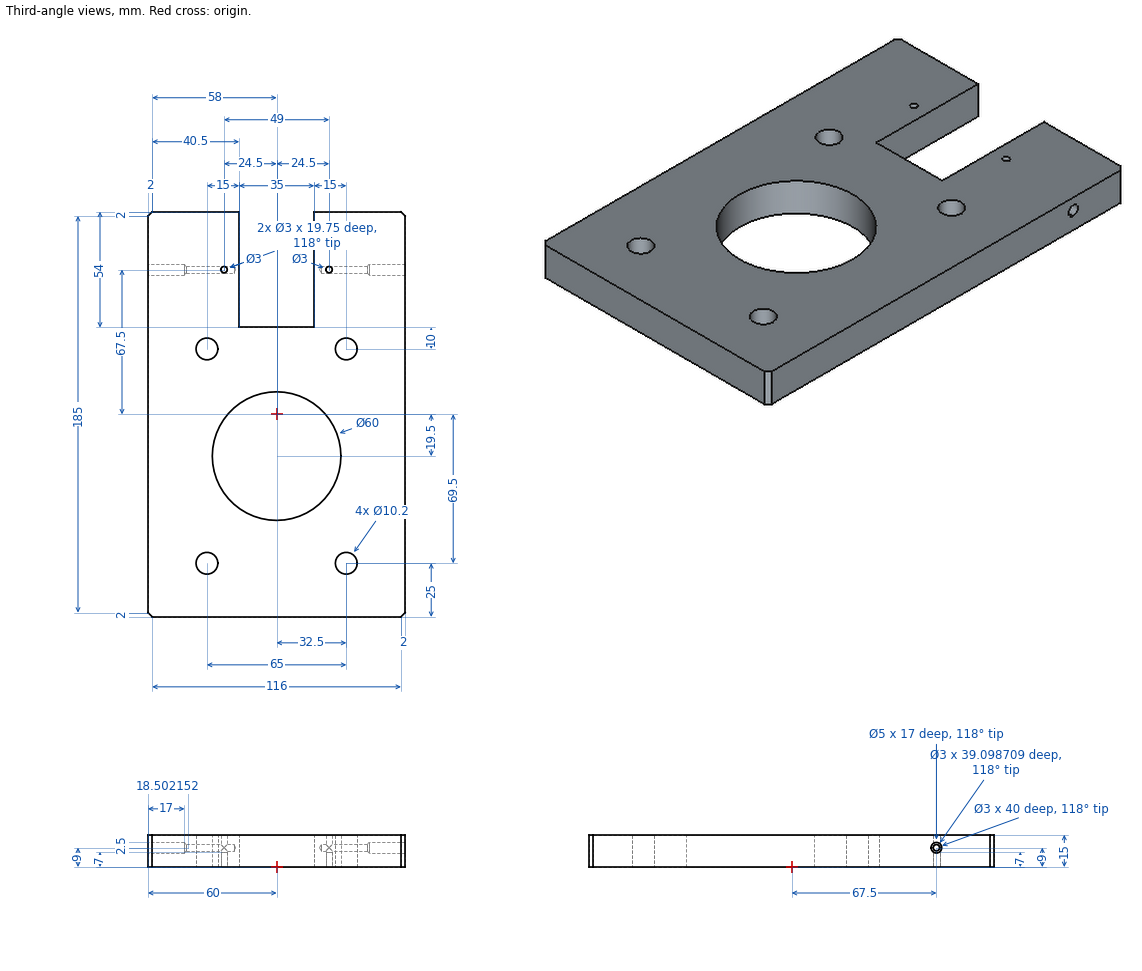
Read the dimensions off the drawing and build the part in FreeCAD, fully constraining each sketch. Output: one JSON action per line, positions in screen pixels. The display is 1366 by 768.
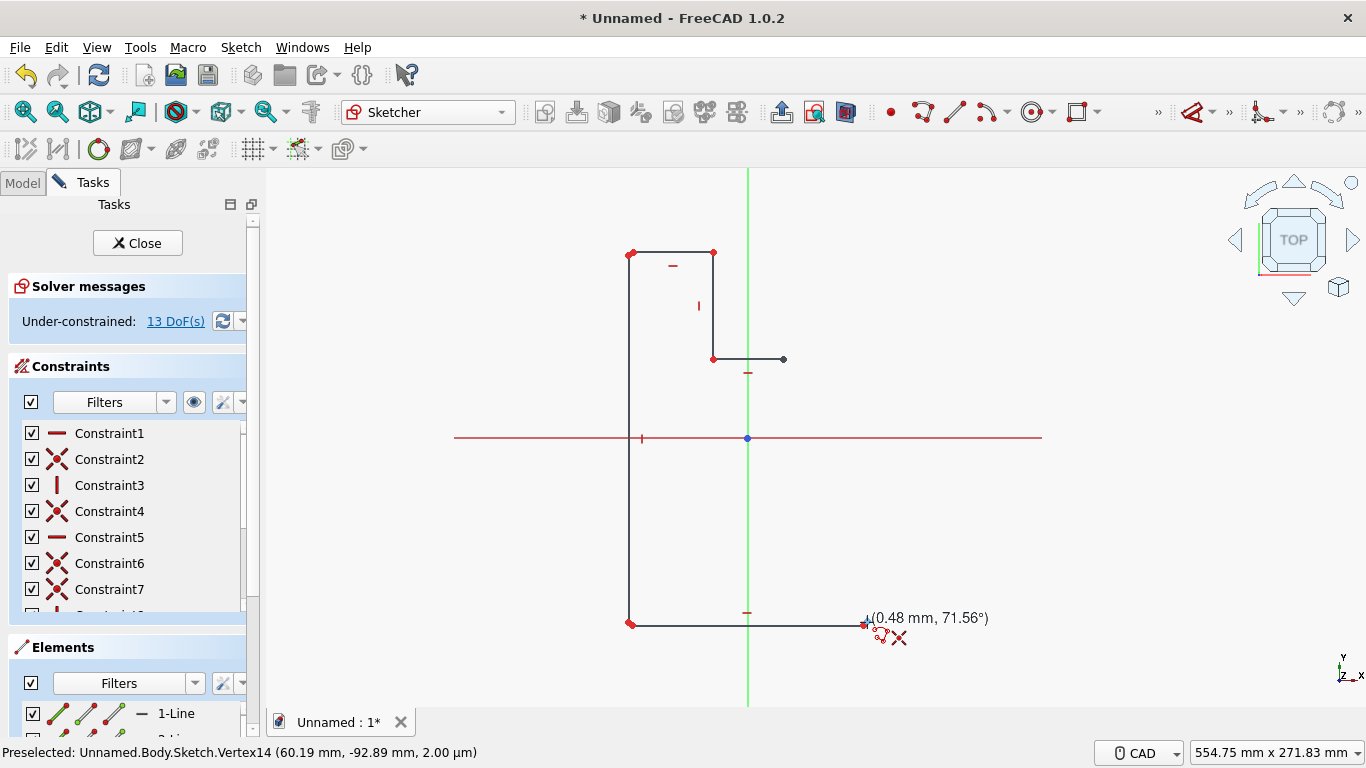
{"action": "left_click", "coordinate": [867, 255]}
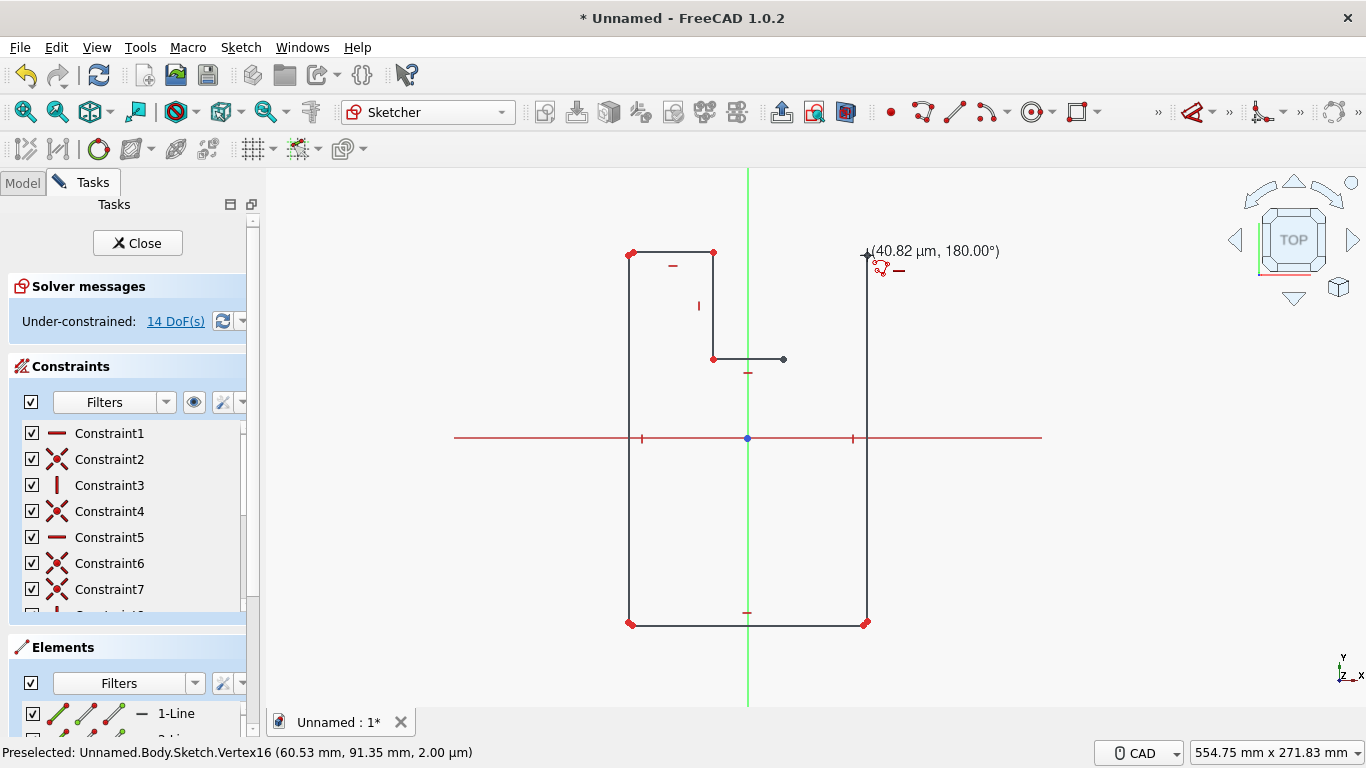
{"action": "scroll", "coordinate": [863, 251], "scroll_direction": "up", "scroll_amount": 6}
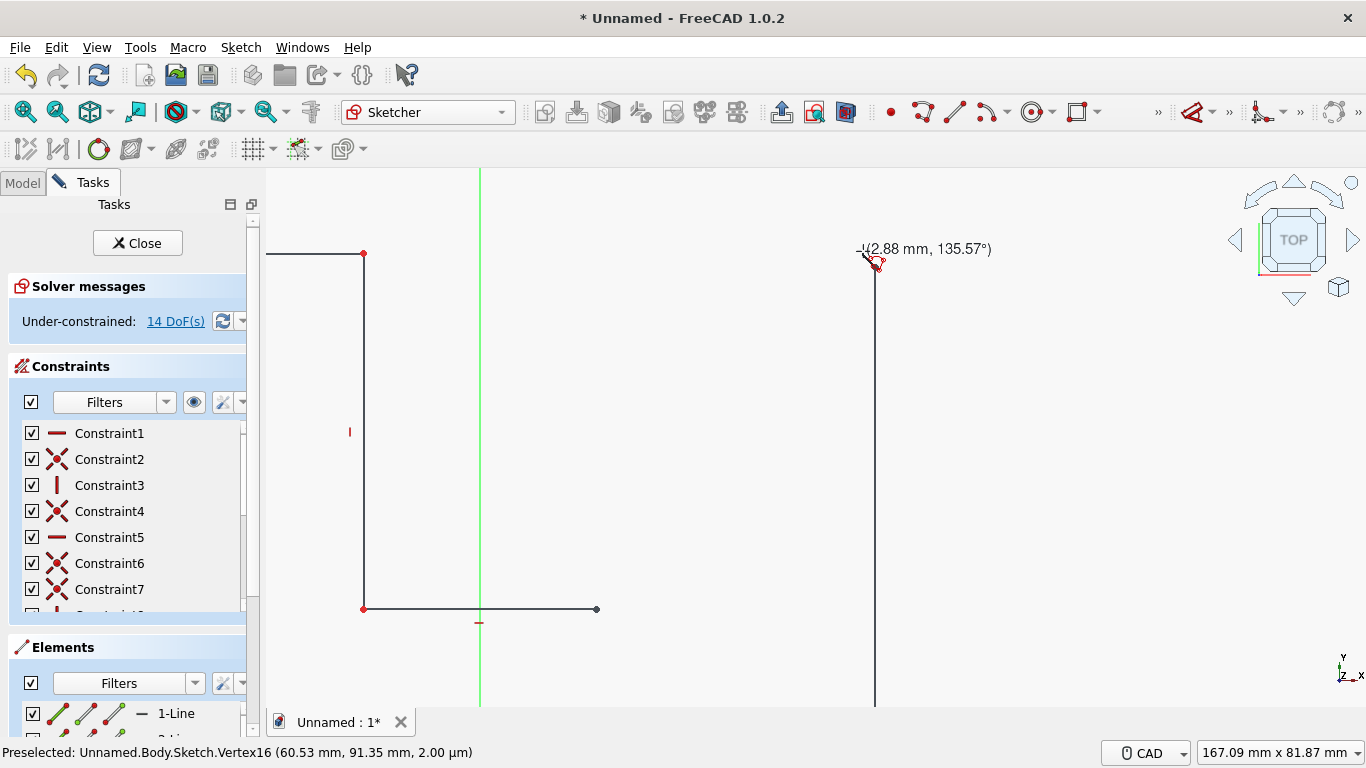
{"action": "left_click", "coordinate": [862, 250]}
{"action": "left_click", "coordinate": [595, 250]}
{"action": "left_click", "coordinate": [596, 609]}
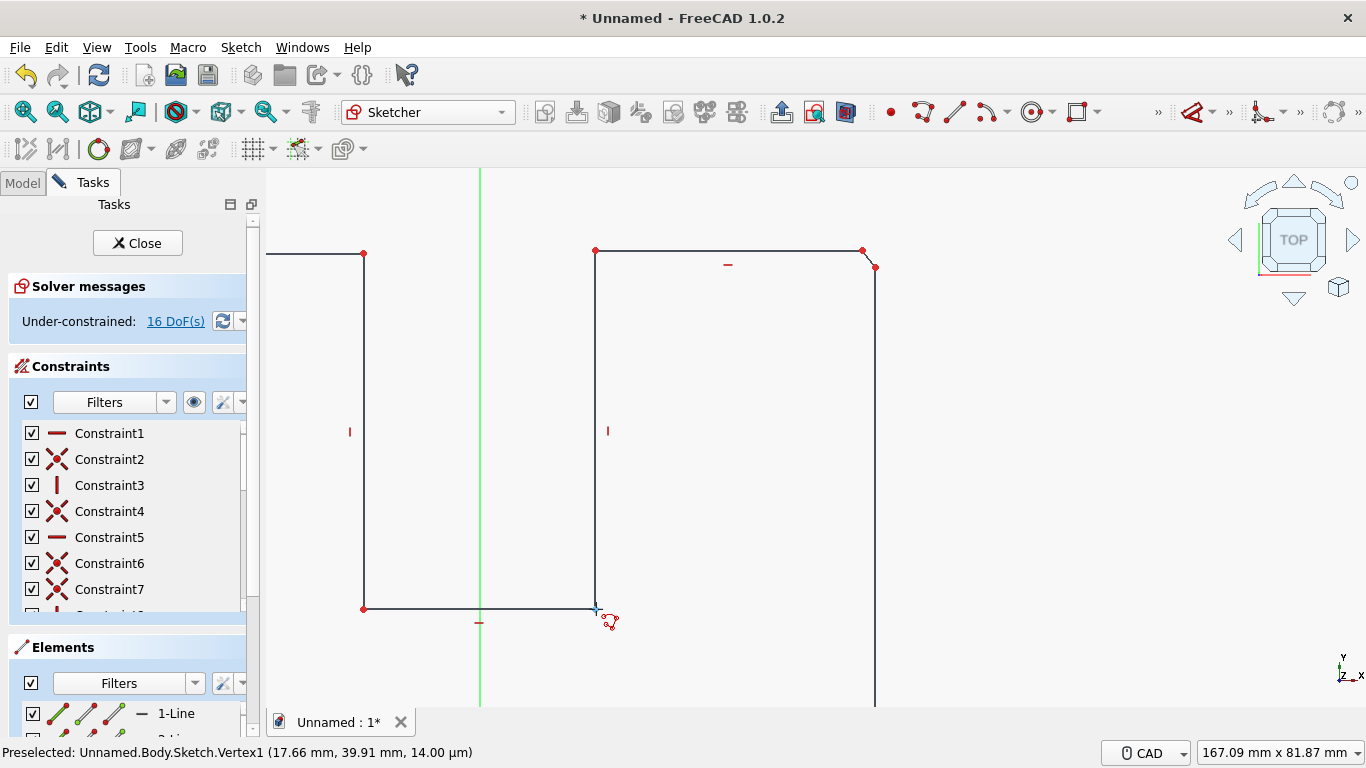
{"action": "left_click", "coordinate": [1032, 112]}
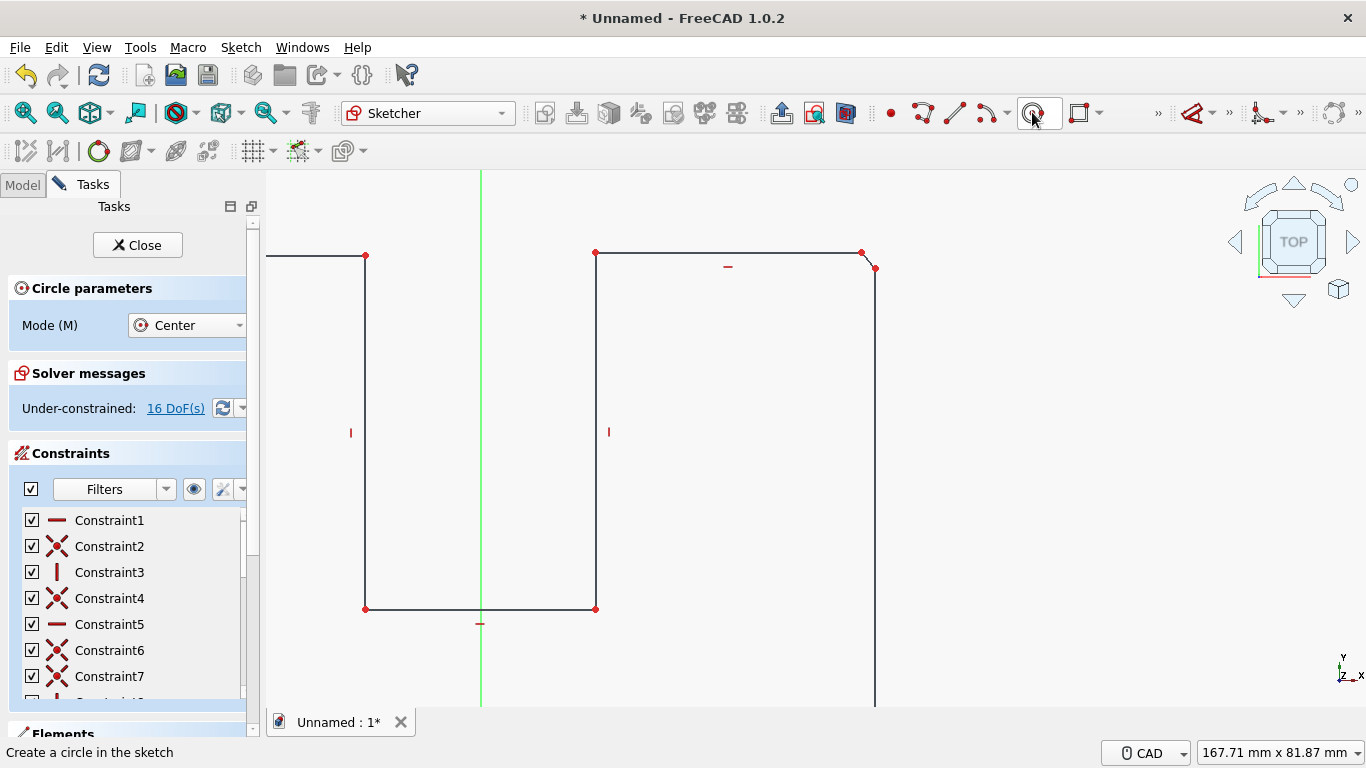
{"action": "scroll", "coordinate": [862, 252], "scroll_direction": "down", "scroll_amount": 6}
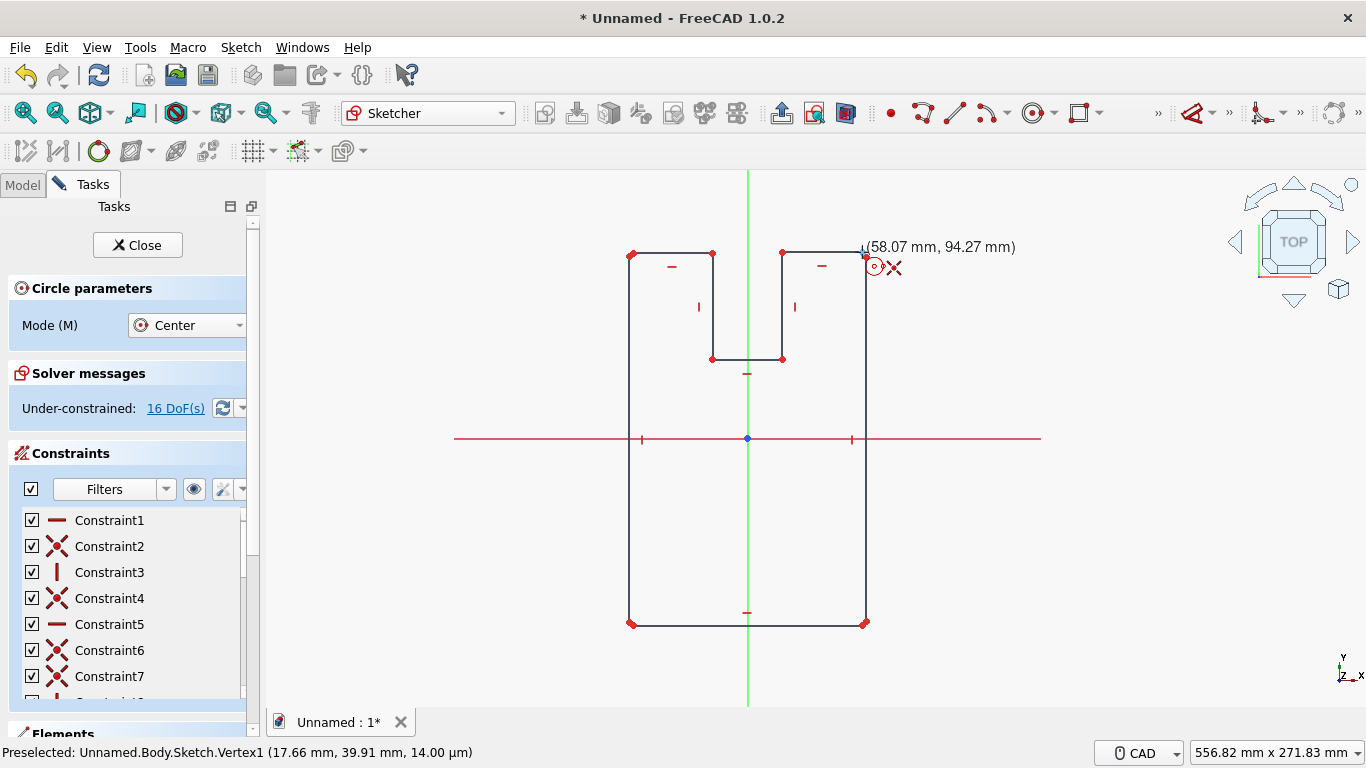
{"action": "scroll", "coordinate": [812, 576], "scroll_direction": "up", "scroll_amount": 5}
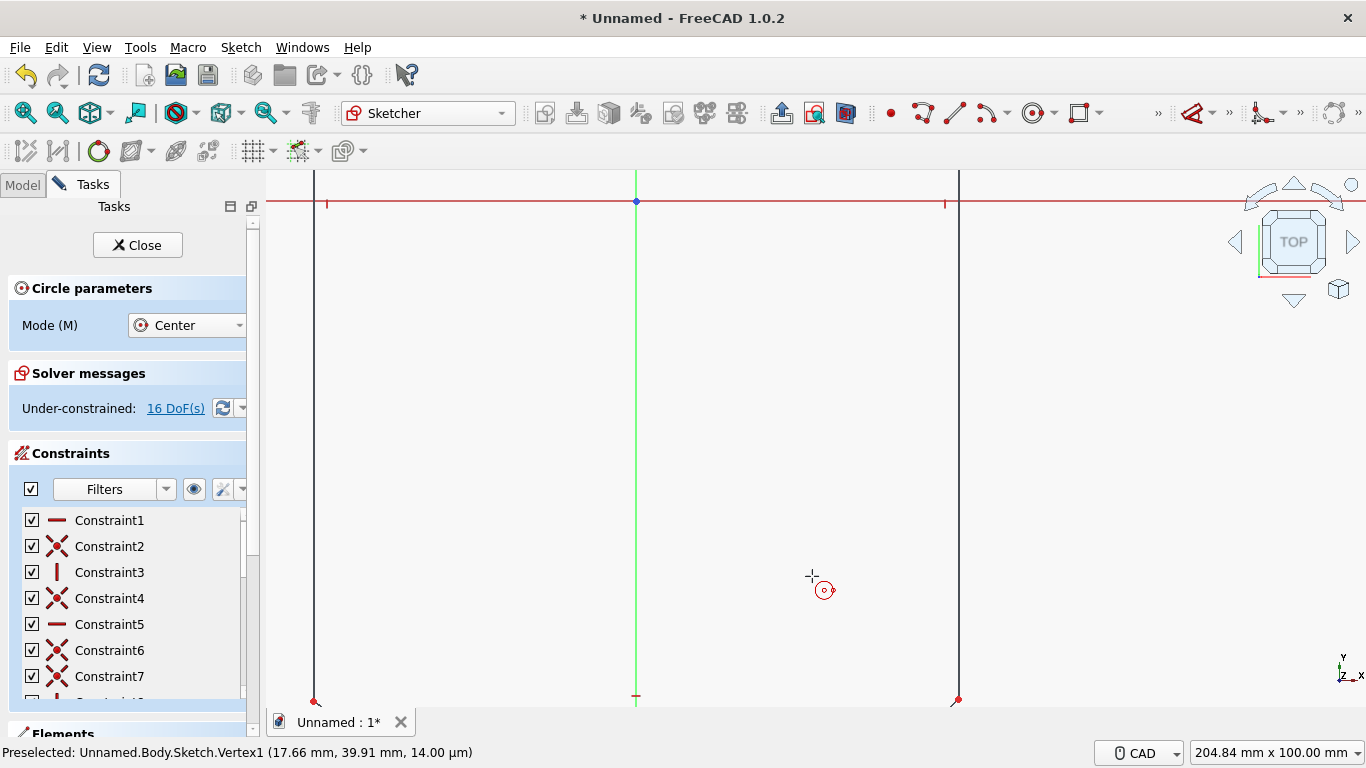
{"action": "left_click", "coordinate": [811, 575]}
{"action": "mouse_move", "coordinate": [830, 555]}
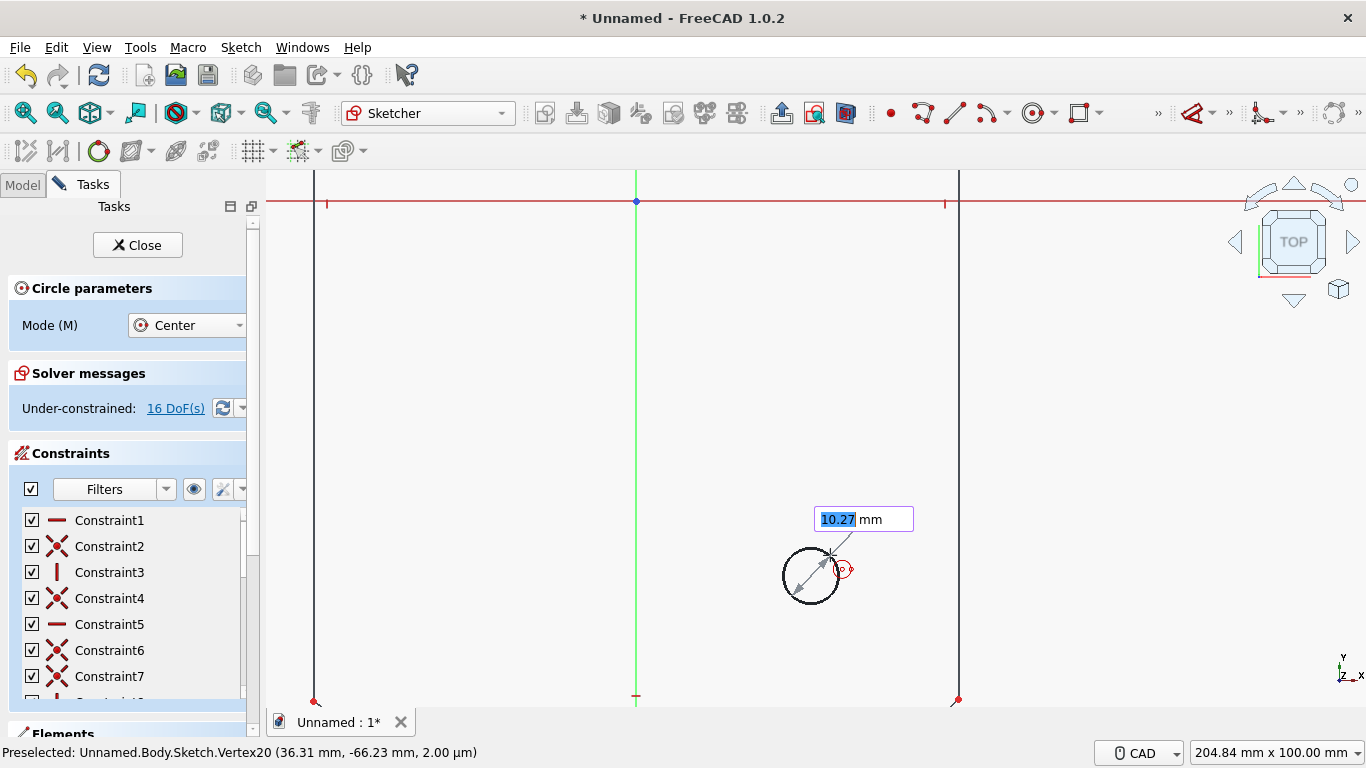
{"action": "type", "text": "10.2"}
{"action": "key", "text": "Return"}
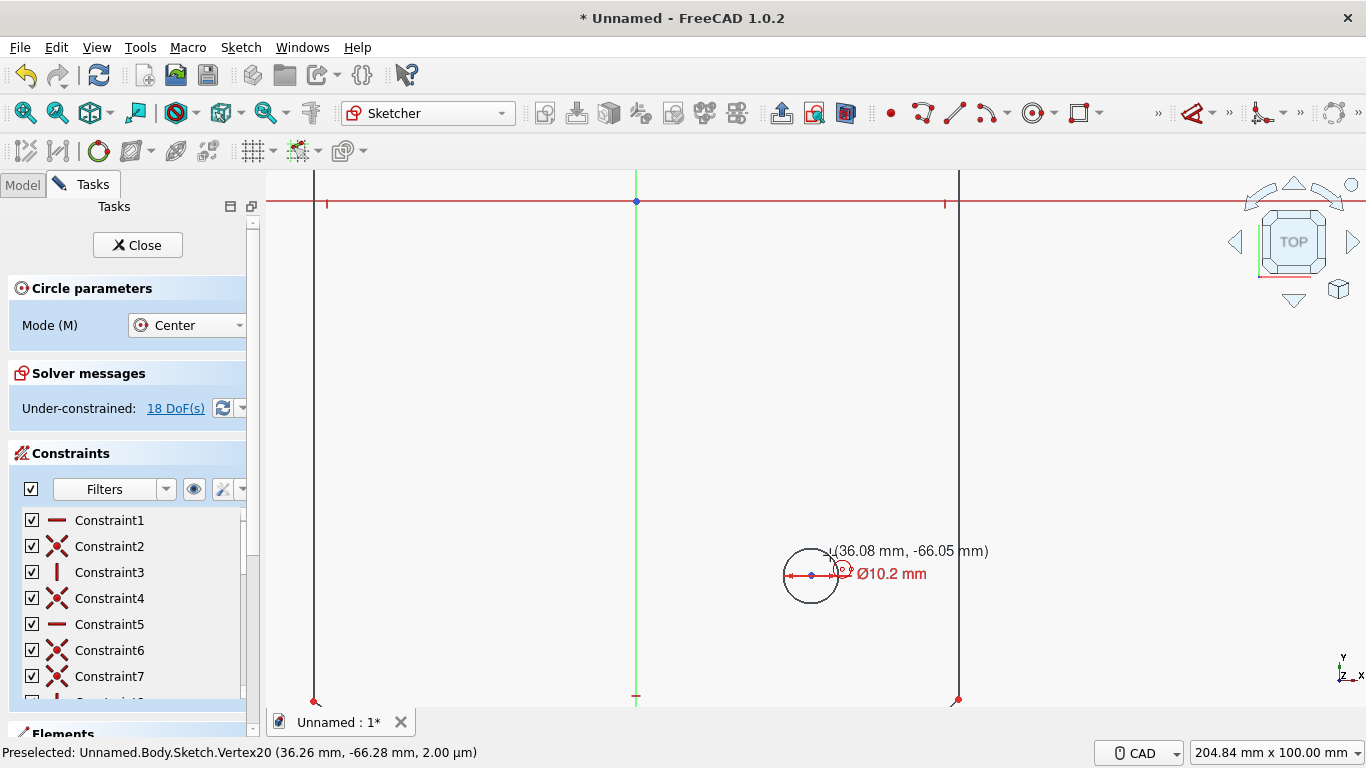
{"action": "left_click", "coordinate": [462, 575]}
{"action": "mouse_move", "coordinate": [481, 555]}